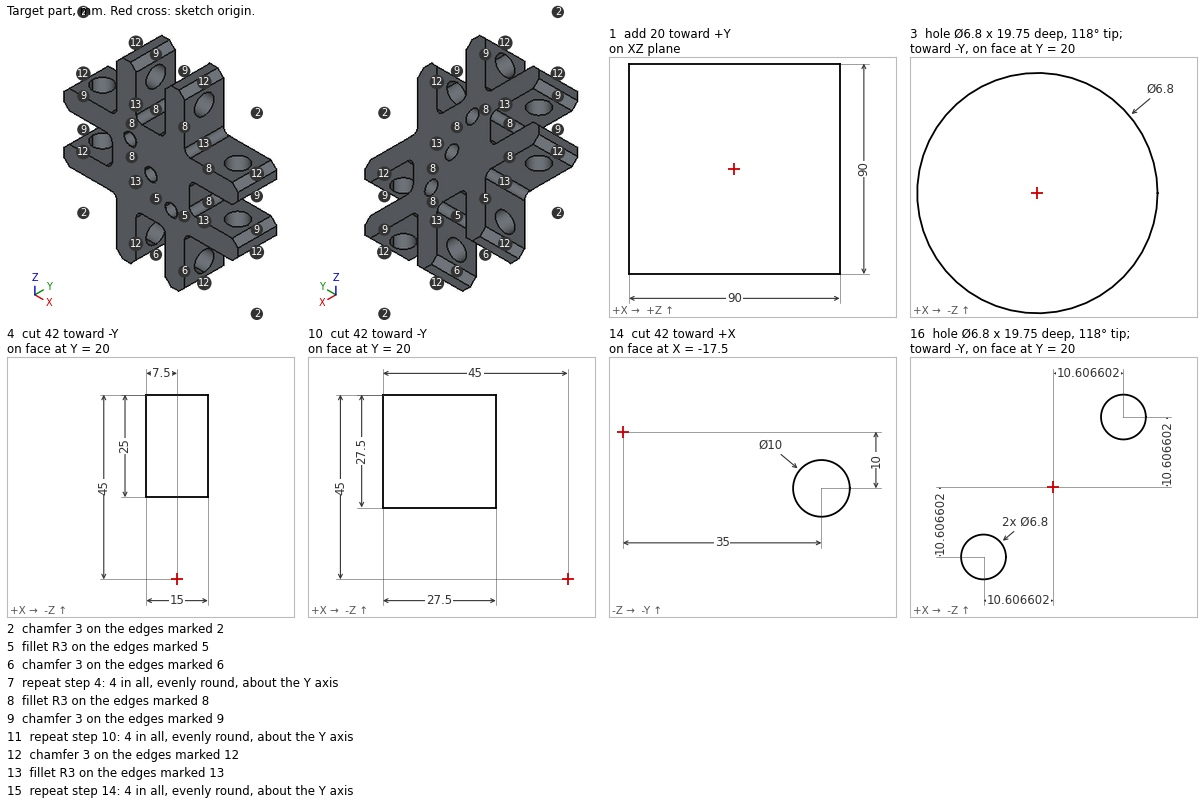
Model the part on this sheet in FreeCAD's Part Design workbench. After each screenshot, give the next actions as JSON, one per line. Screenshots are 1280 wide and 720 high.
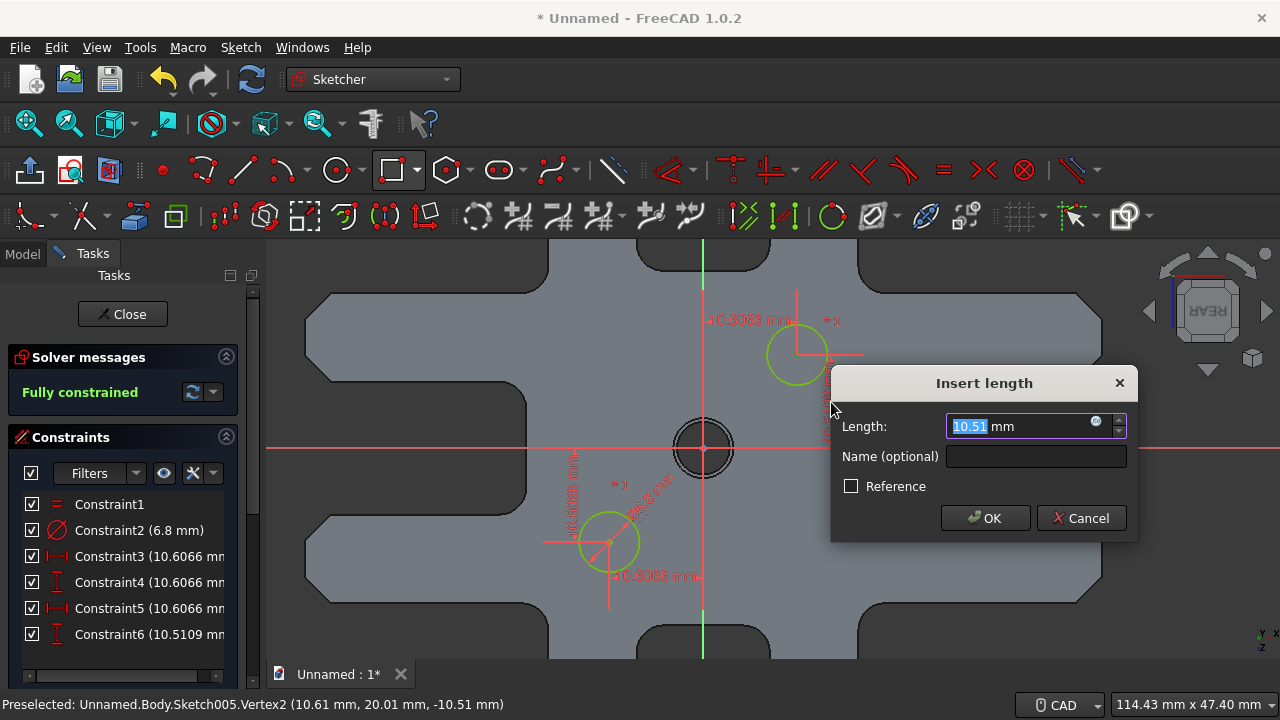
{"action": "type", "text": "10.606602"}
{"action": "key", "text": "Return"}
{"action": "key", "text": "Escape"}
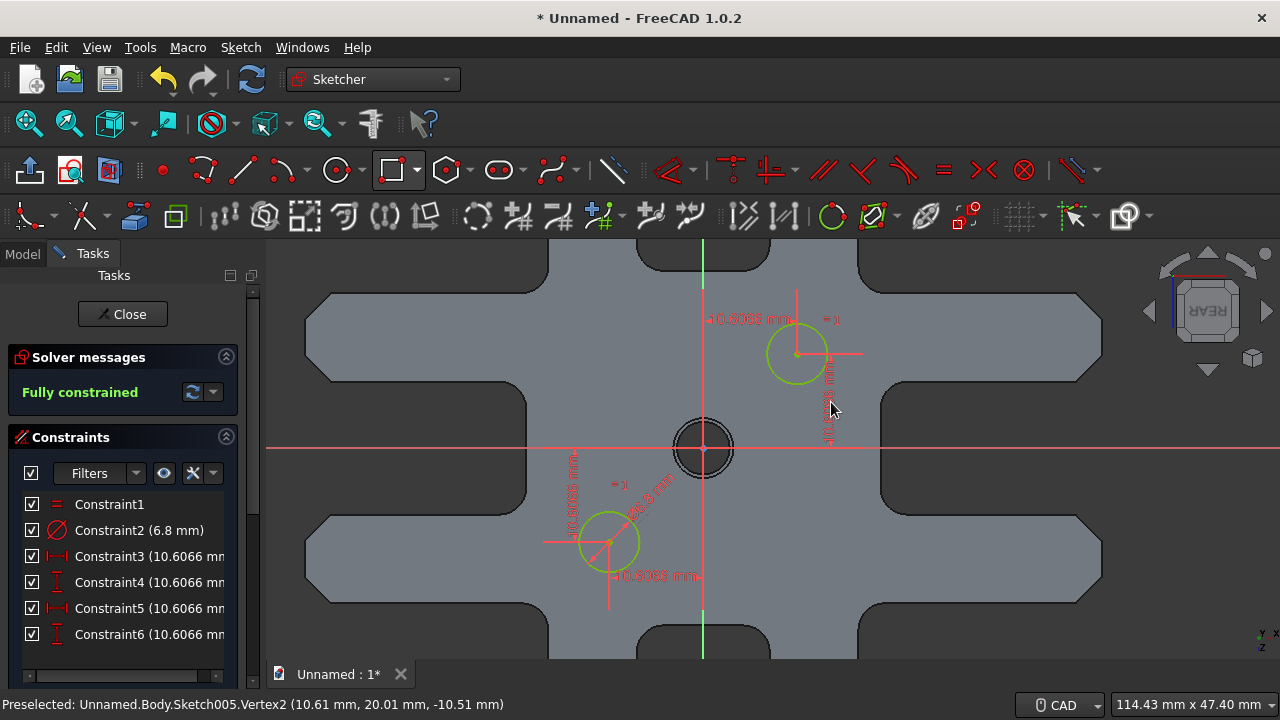
{"action": "left_click", "coordinate": [123, 314]}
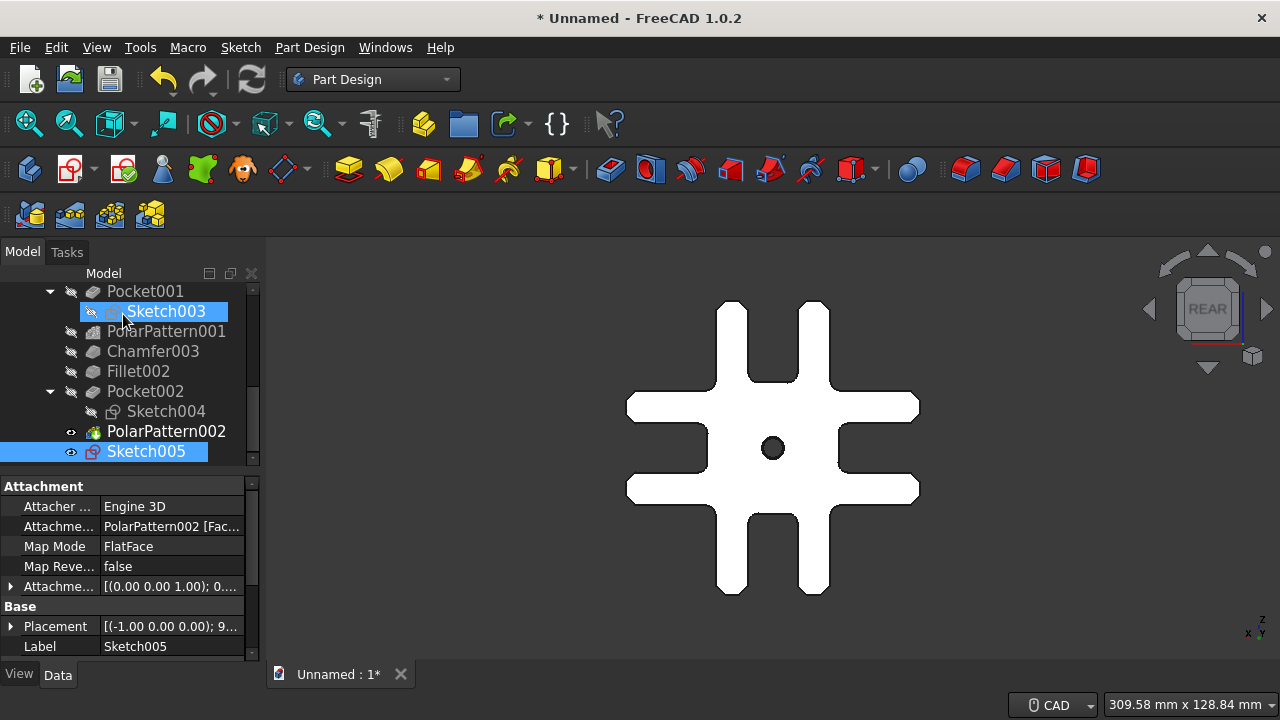
{"action": "left_click", "coordinate": [652, 170]}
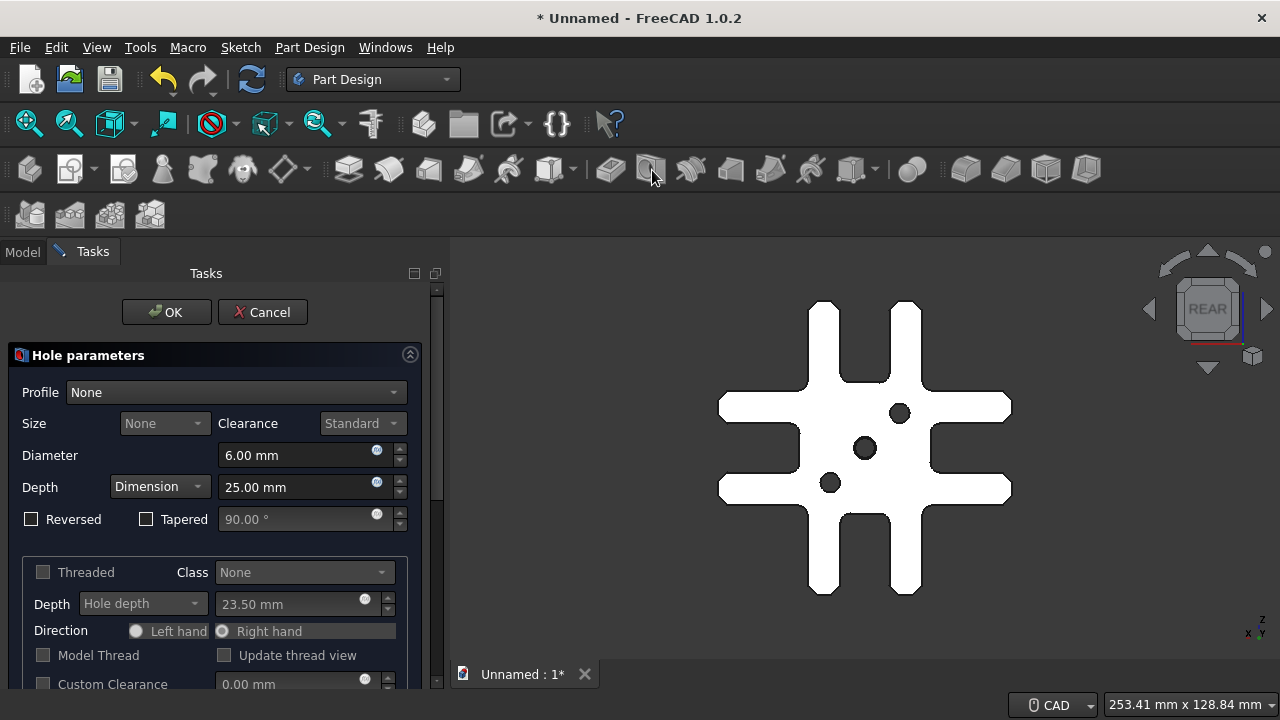
{"action": "triple_click", "coordinate": [305, 455]}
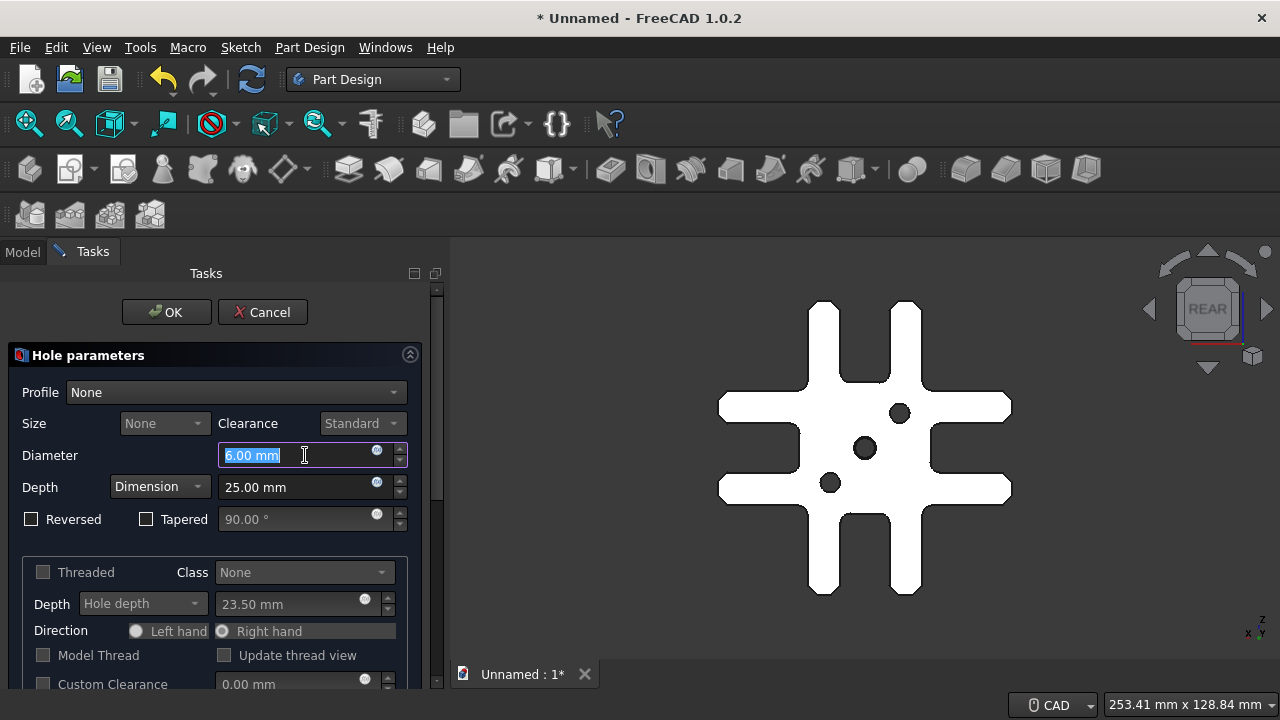
{"action": "type", "text": "6.8"}
{"action": "key", "text": "Tab"}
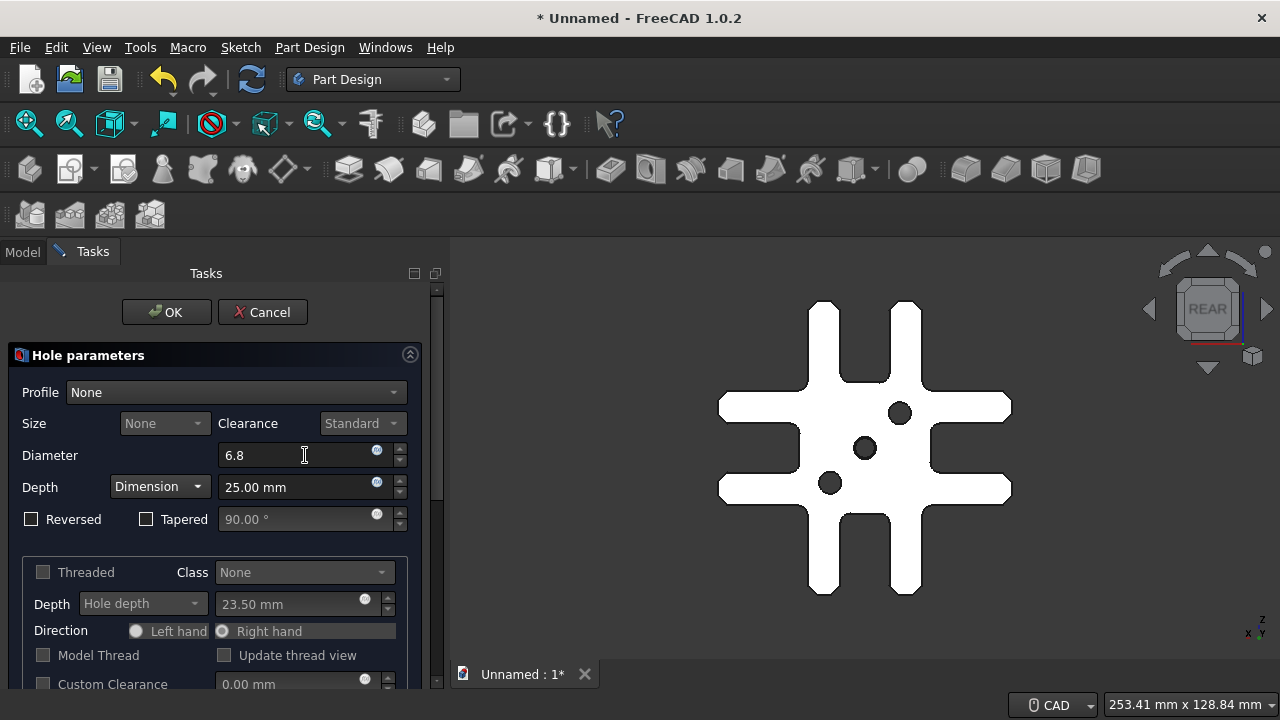
{"action": "triple_click", "coordinate": [305, 487]}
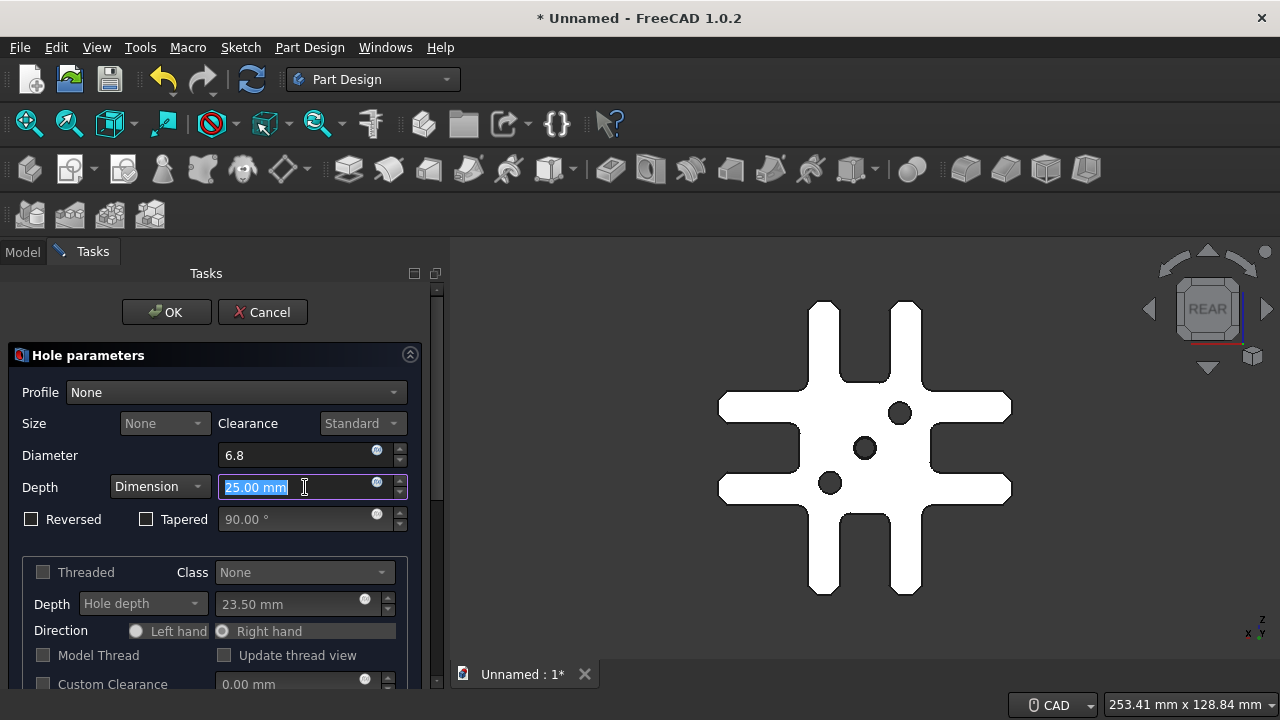
{"action": "type", "text": "19.75"}
{"action": "key", "text": "Tab"}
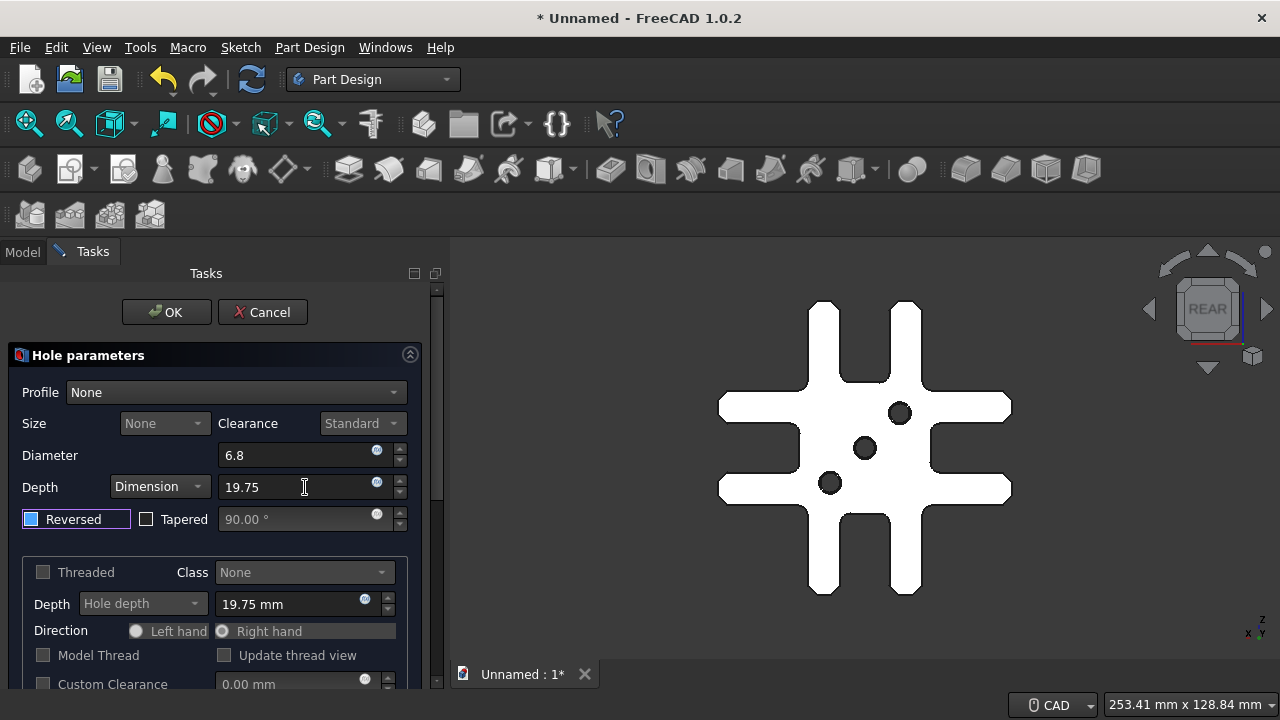
{"action": "left_click", "coordinate": [167, 312]}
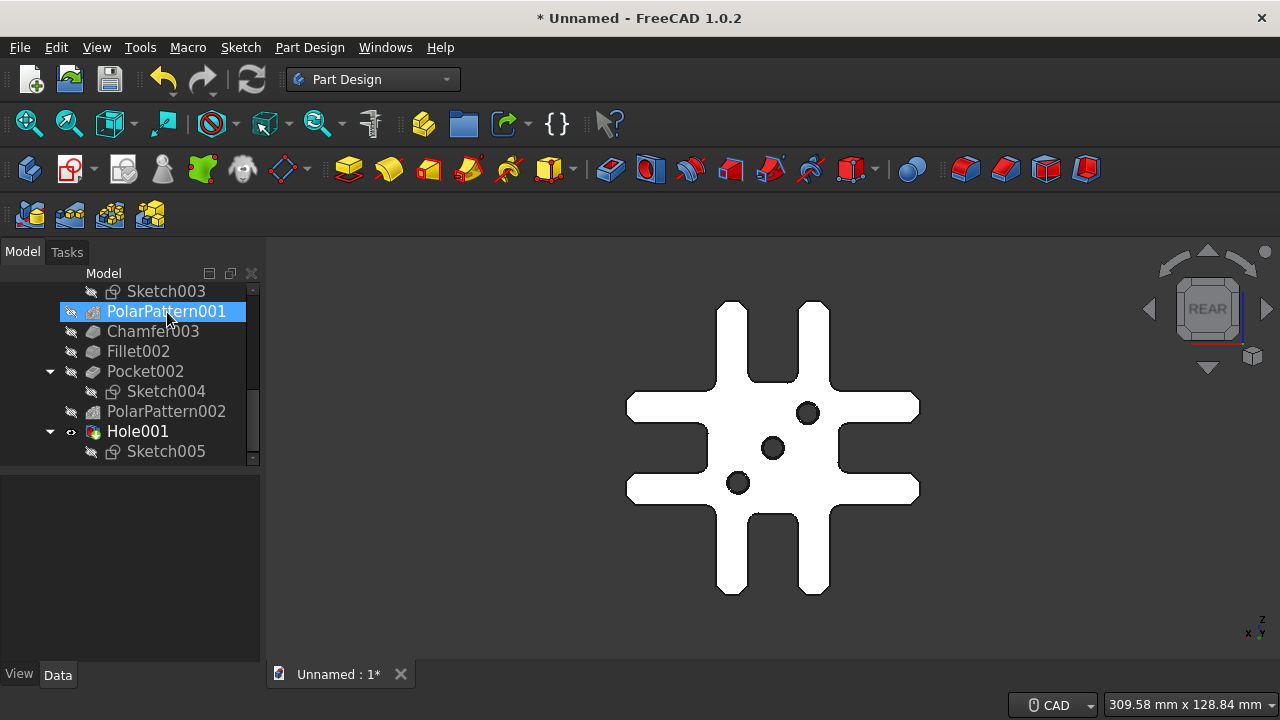
{"action": "key", "text": "0"}